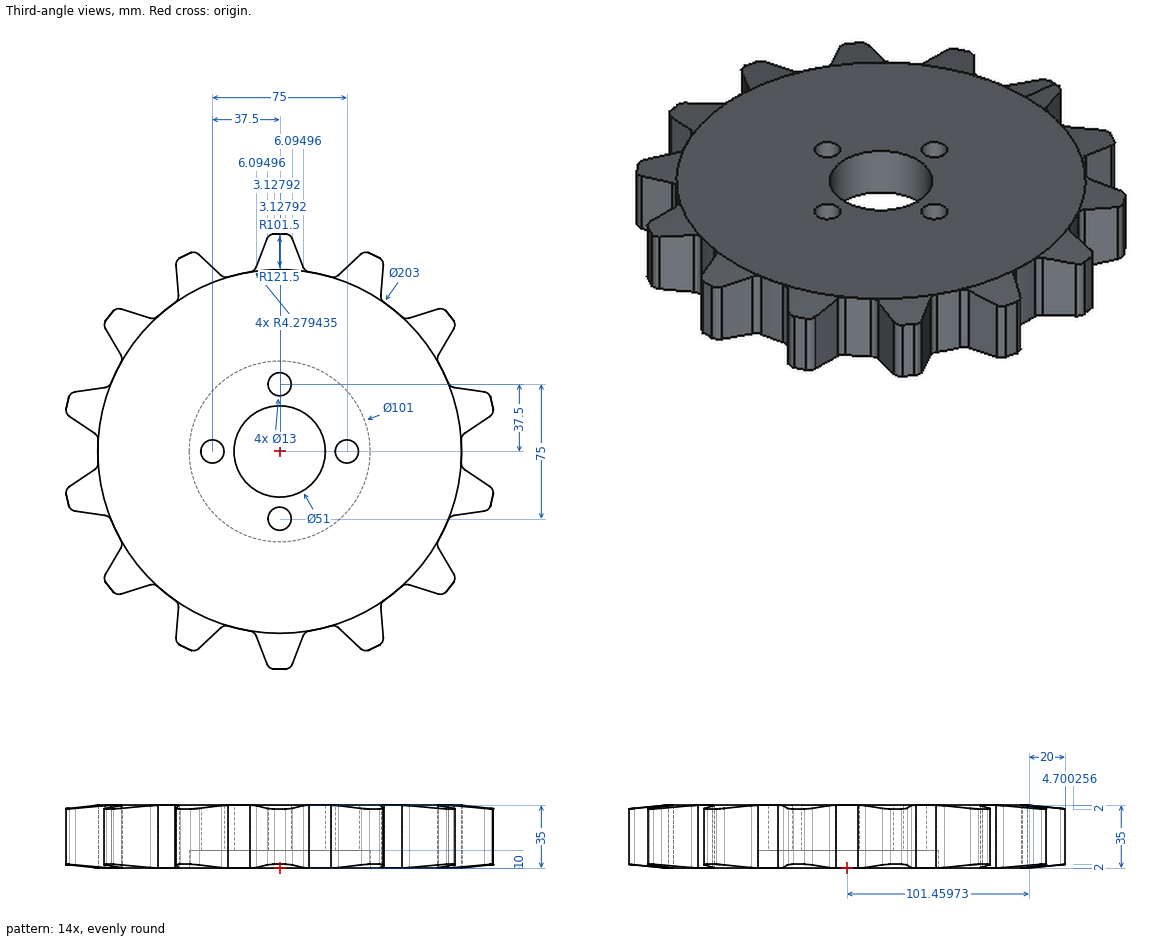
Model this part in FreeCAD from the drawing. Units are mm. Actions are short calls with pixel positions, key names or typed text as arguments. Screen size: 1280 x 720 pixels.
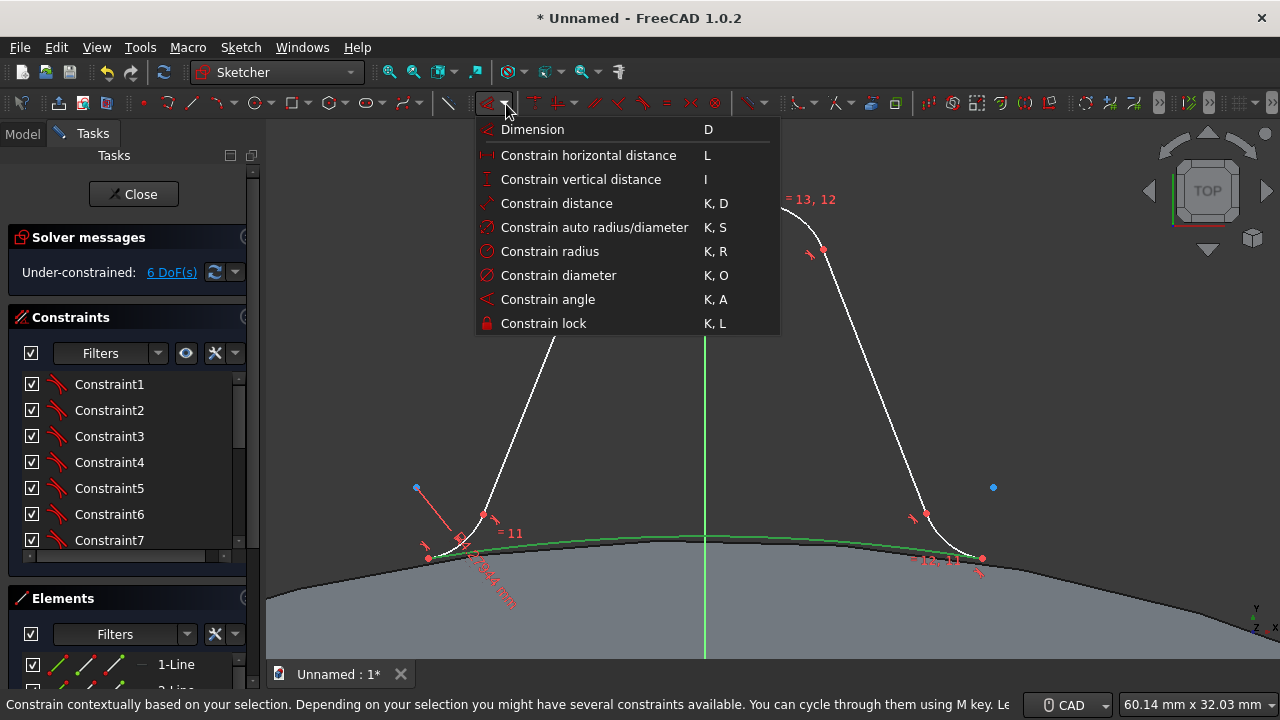
click(628, 251)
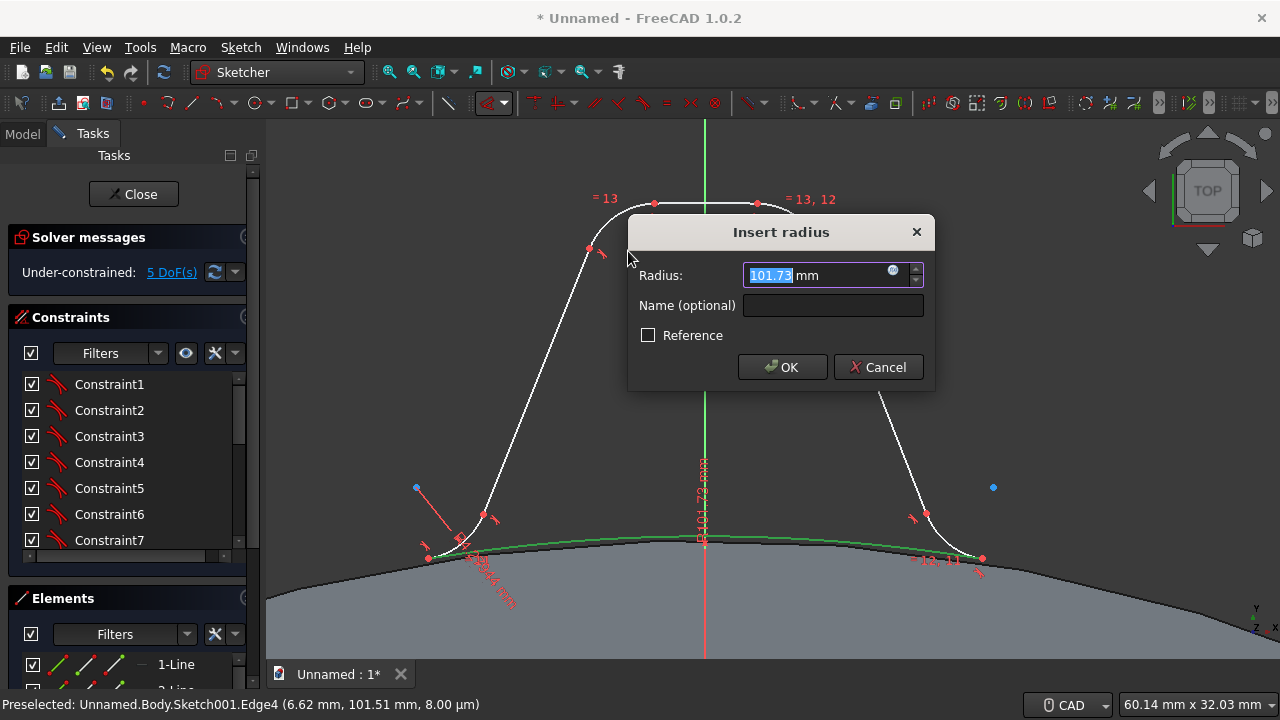
text(101.5)
key(Return)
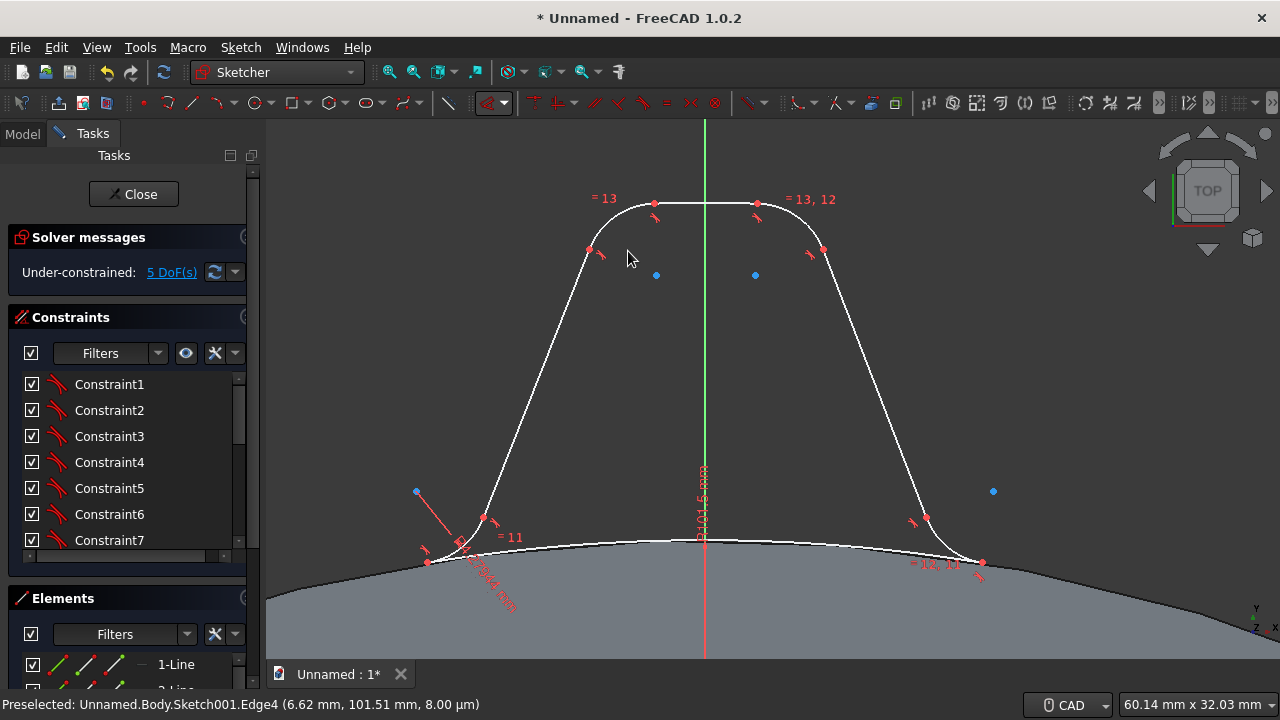
click(727, 203)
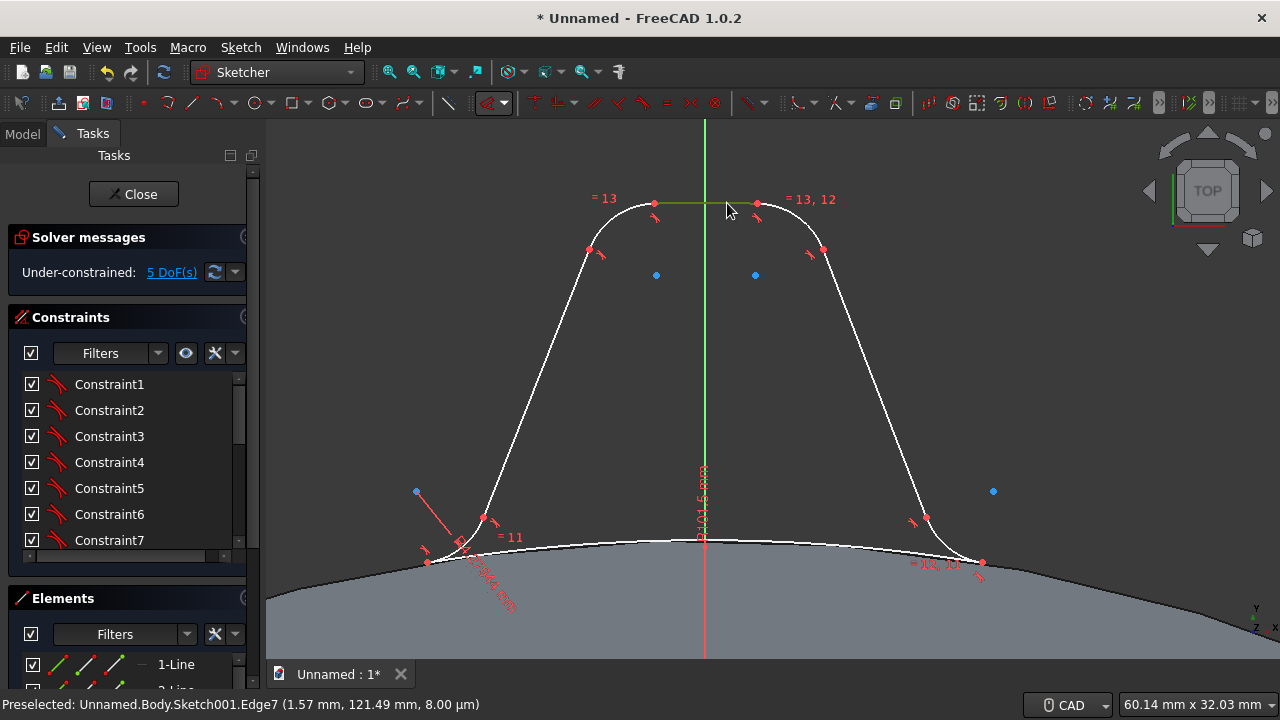
click(506, 104)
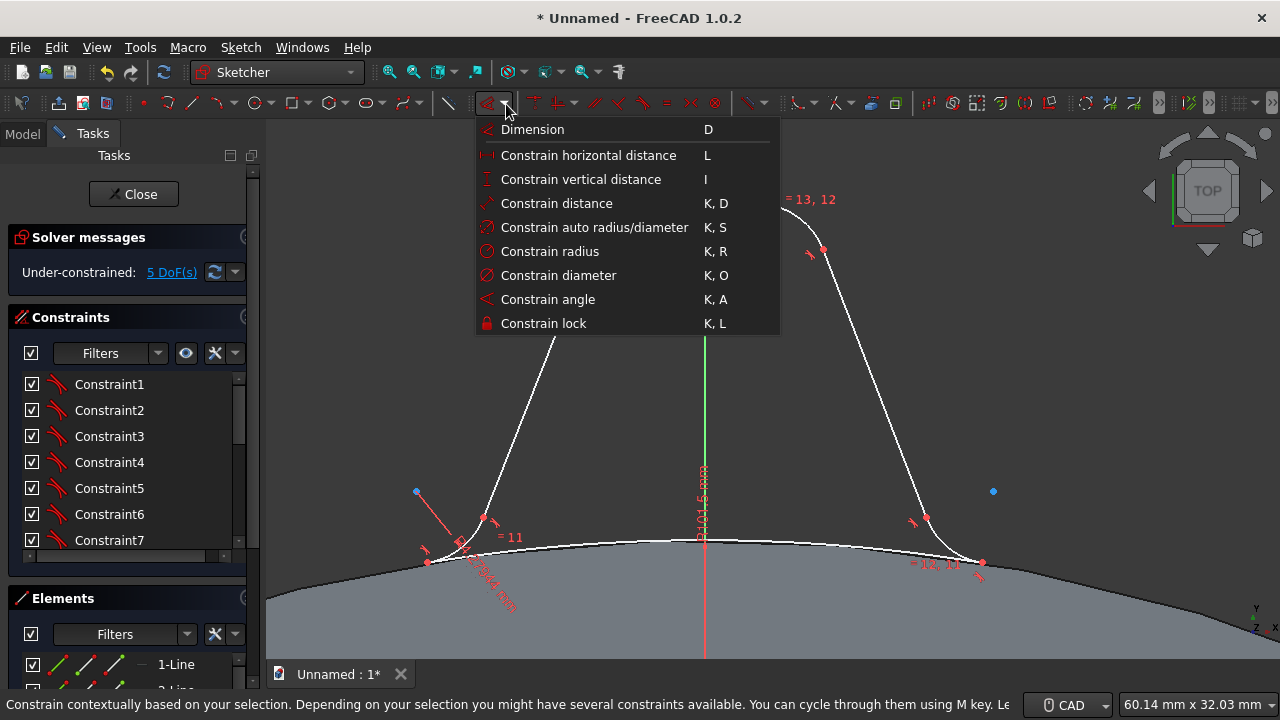
click(628, 251)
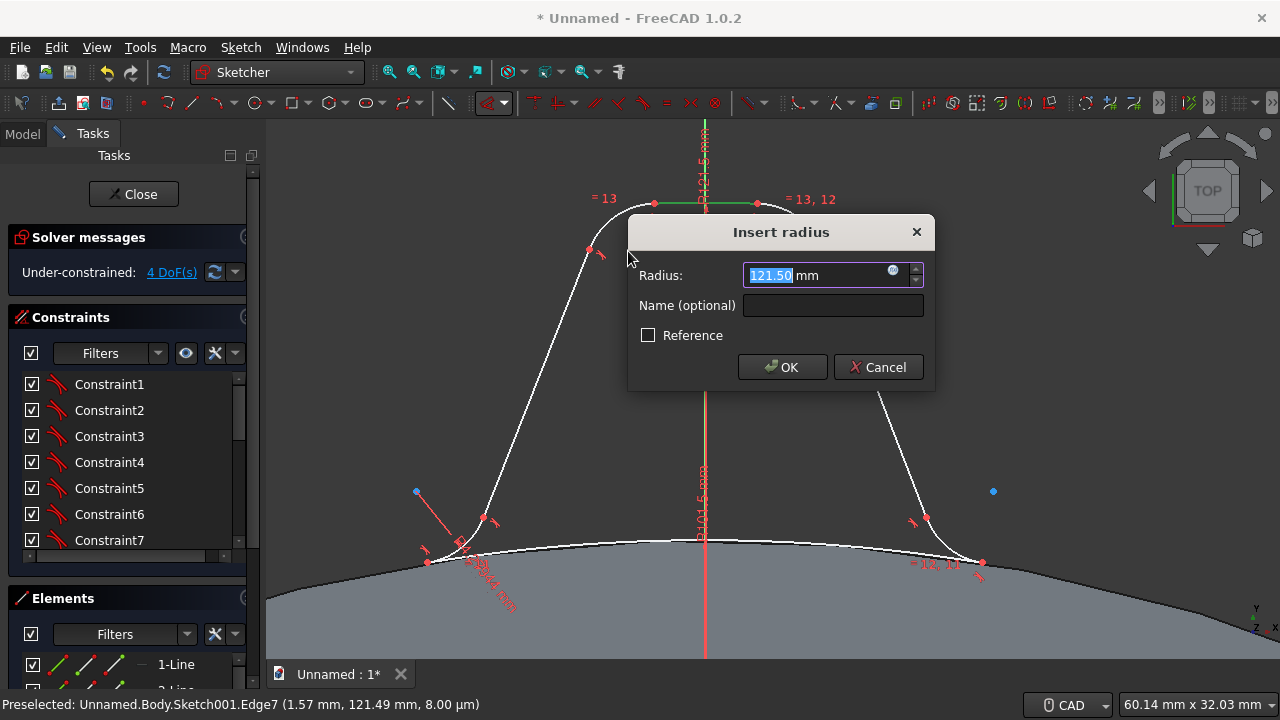
text(121.5)
key(Return)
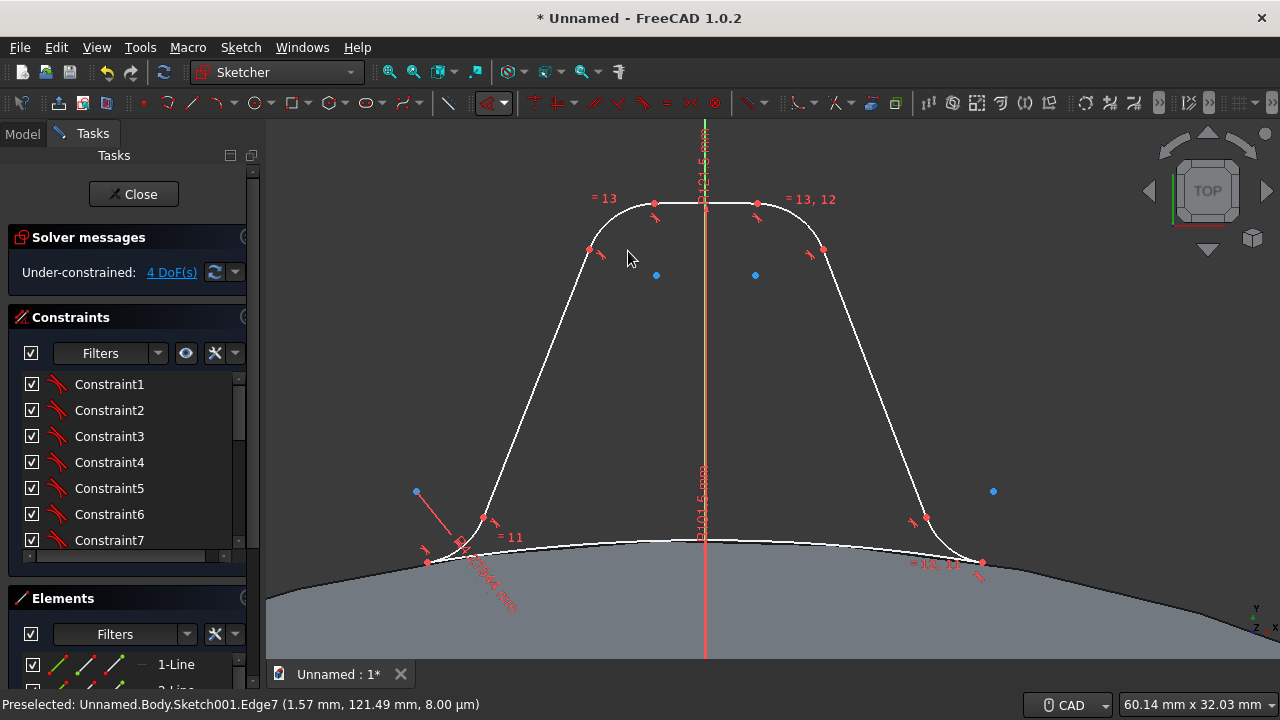
click(758, 204)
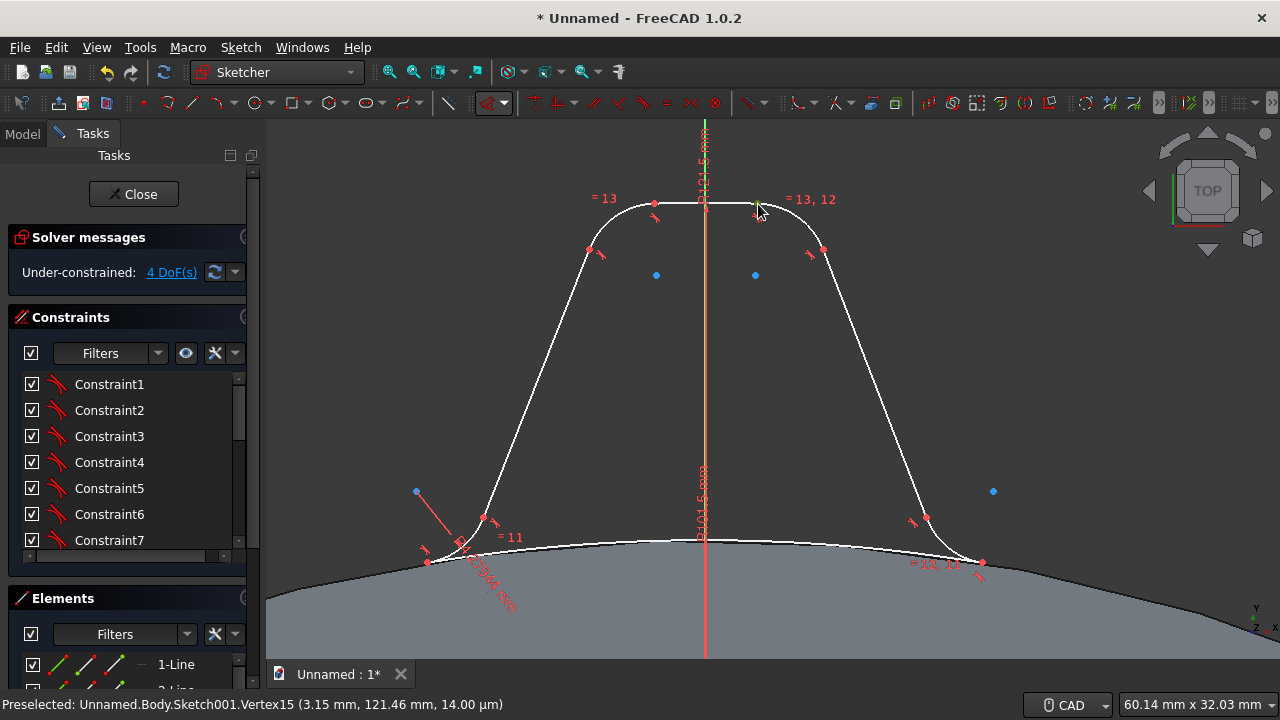
key(l)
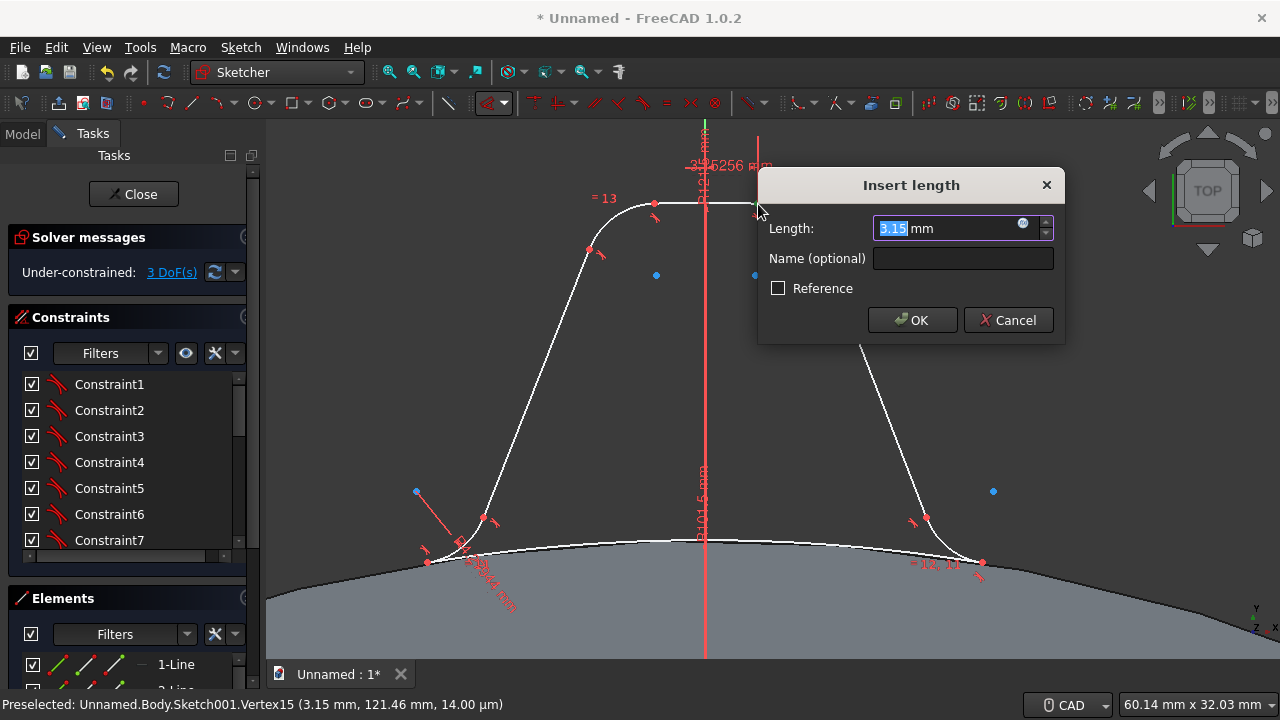
text(3.12792)
key(Return)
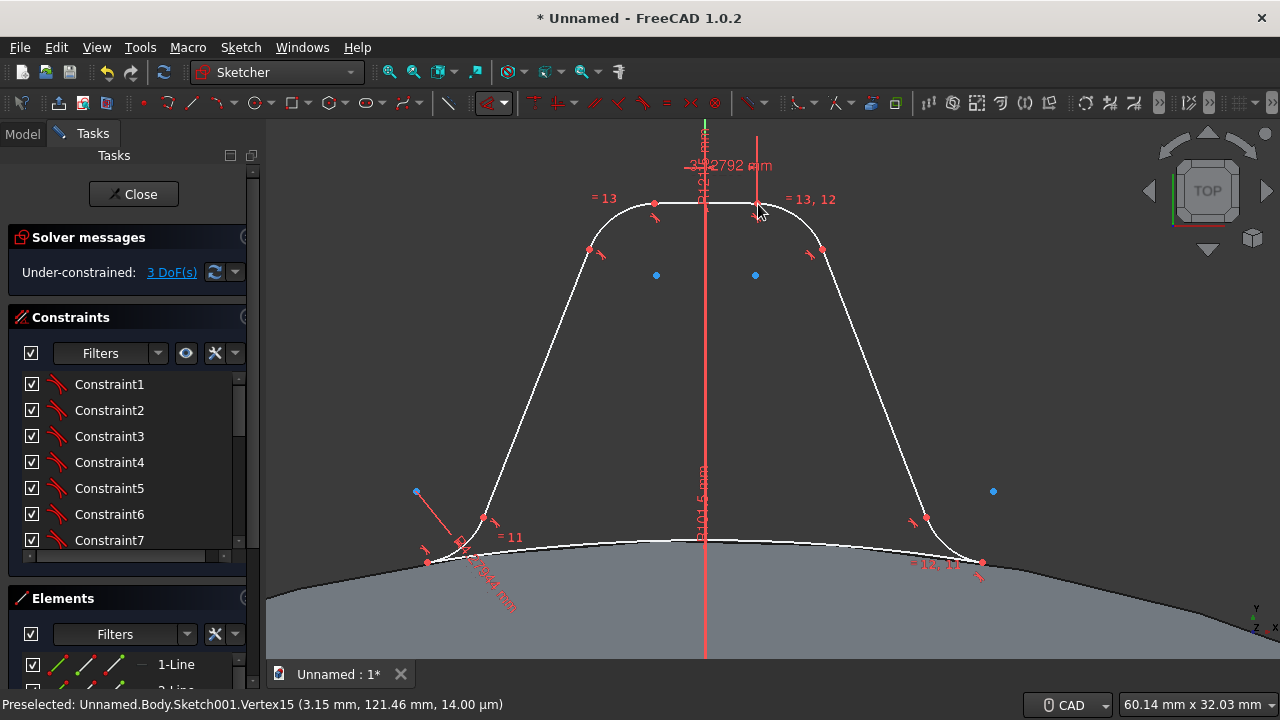
click(655, 204)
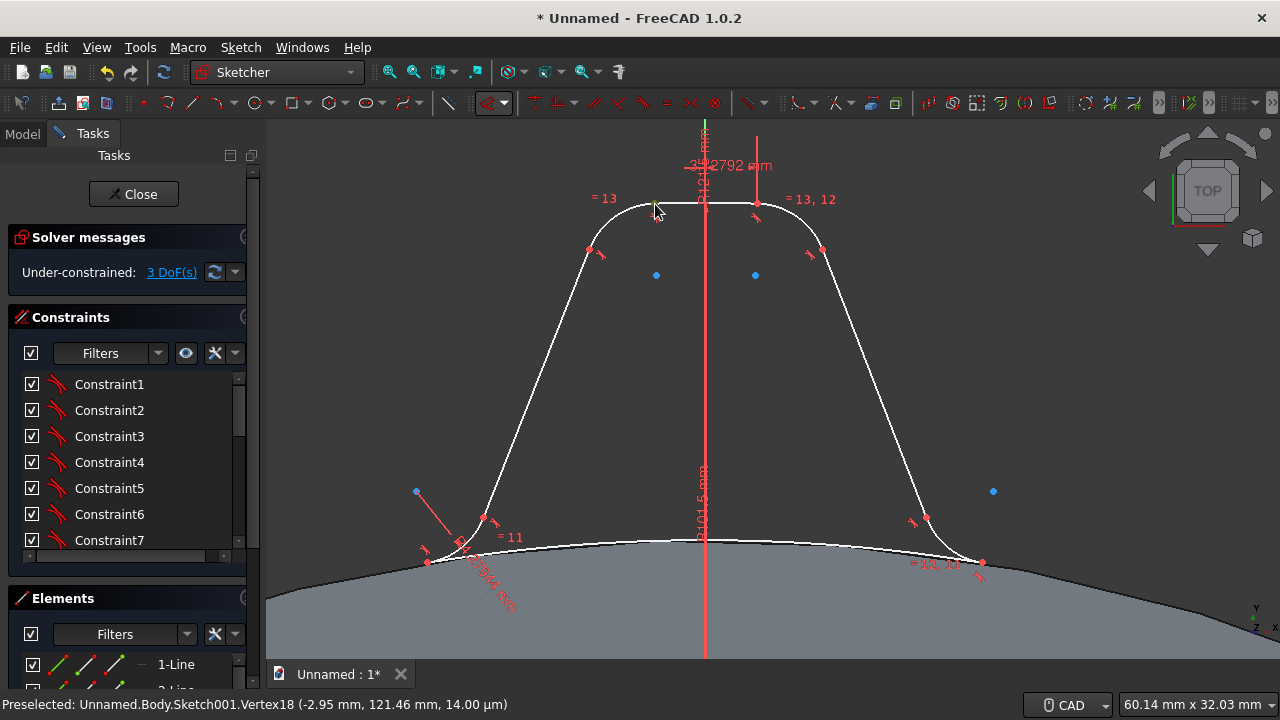
key(l)